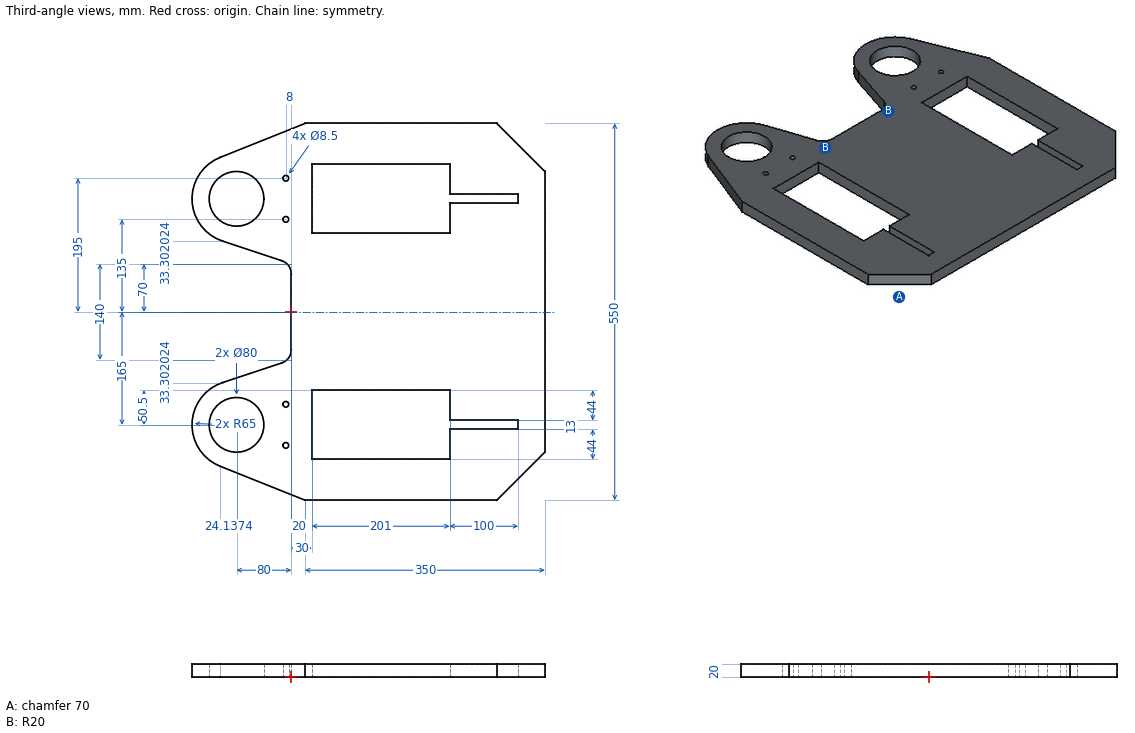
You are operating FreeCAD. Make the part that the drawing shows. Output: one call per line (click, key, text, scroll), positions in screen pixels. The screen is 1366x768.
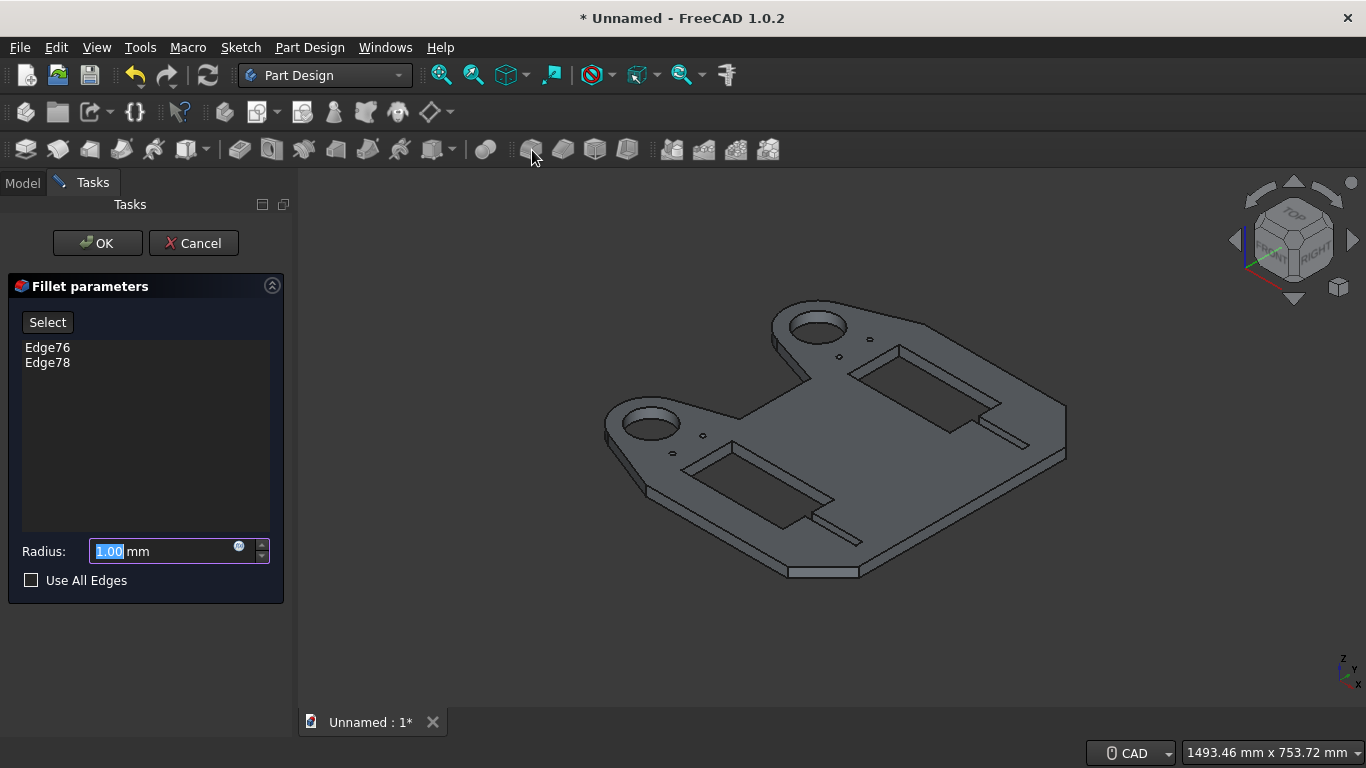
text(20)
key(Tab)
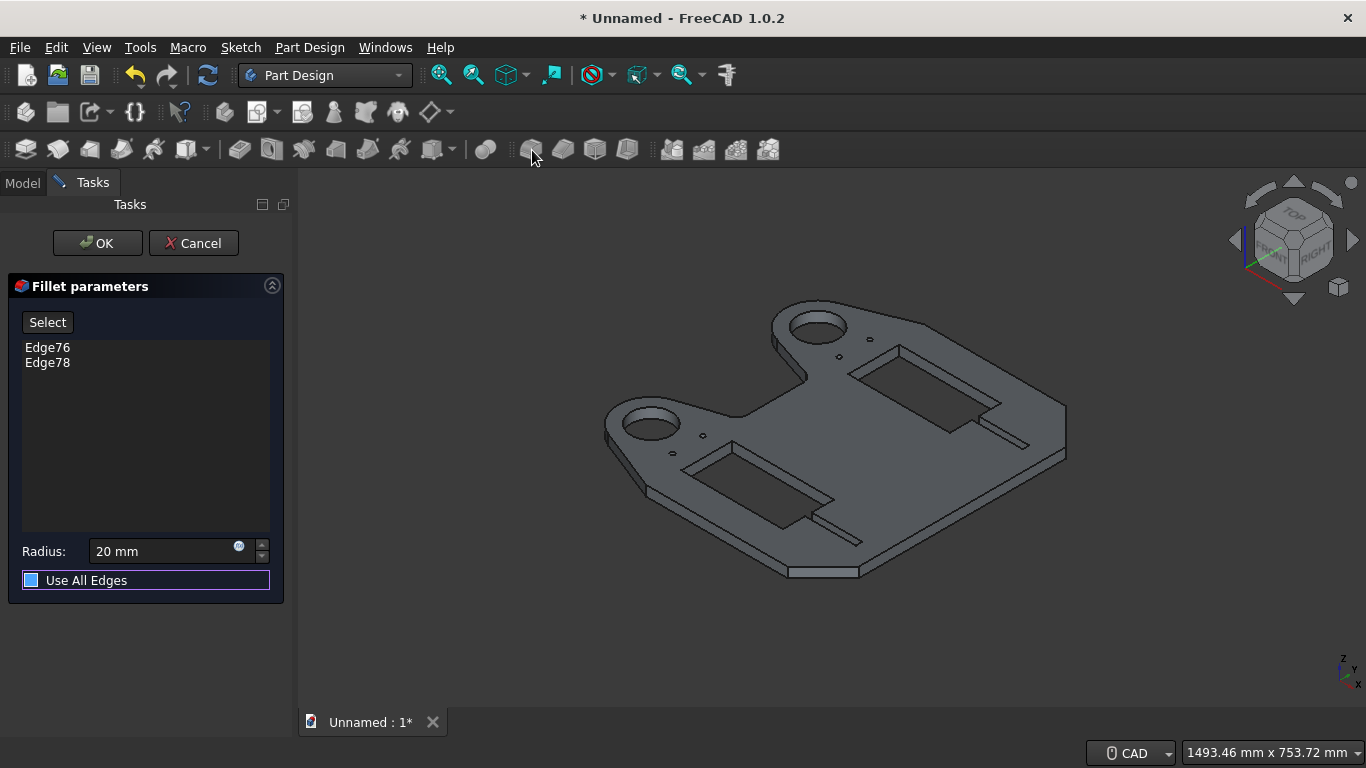
click(98, 243)